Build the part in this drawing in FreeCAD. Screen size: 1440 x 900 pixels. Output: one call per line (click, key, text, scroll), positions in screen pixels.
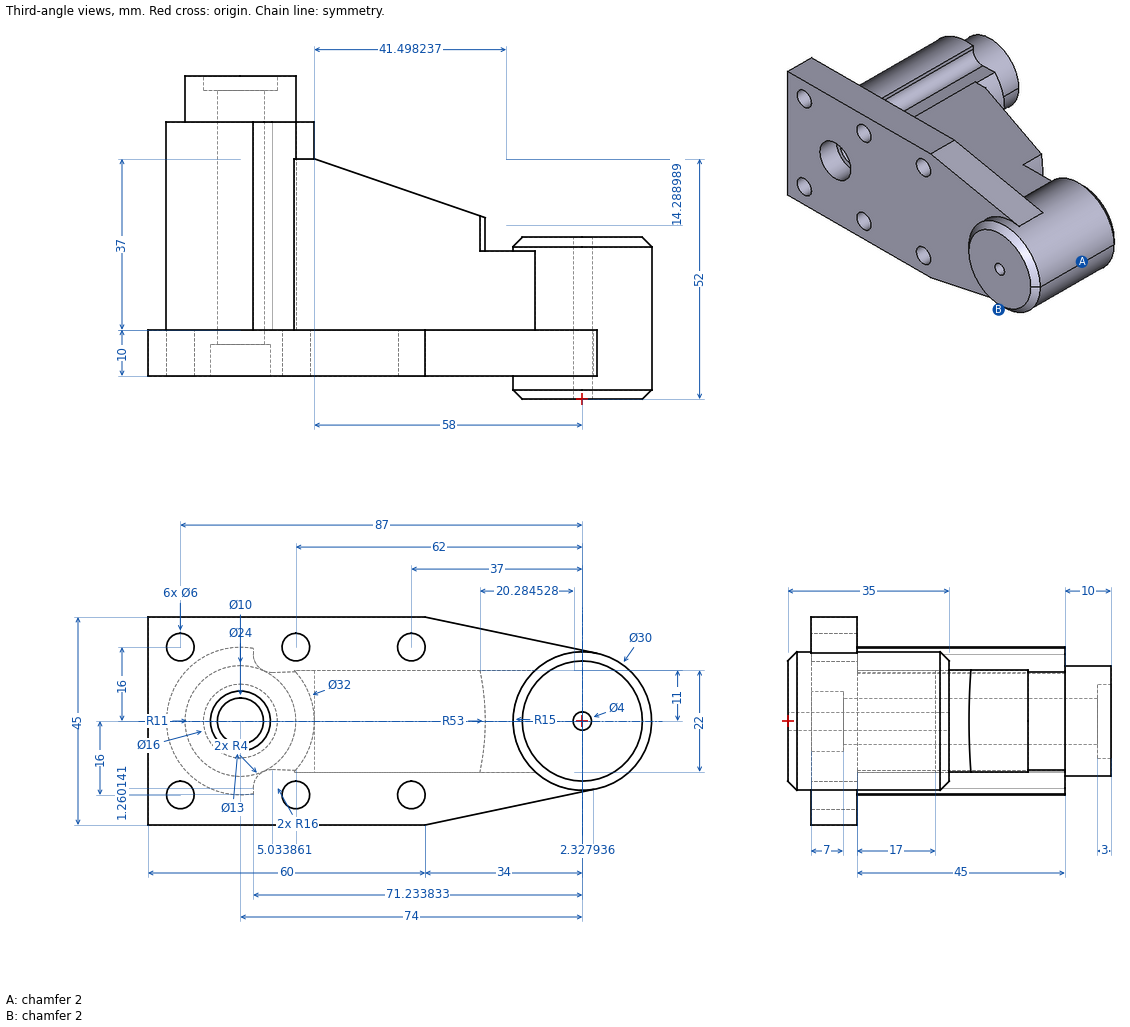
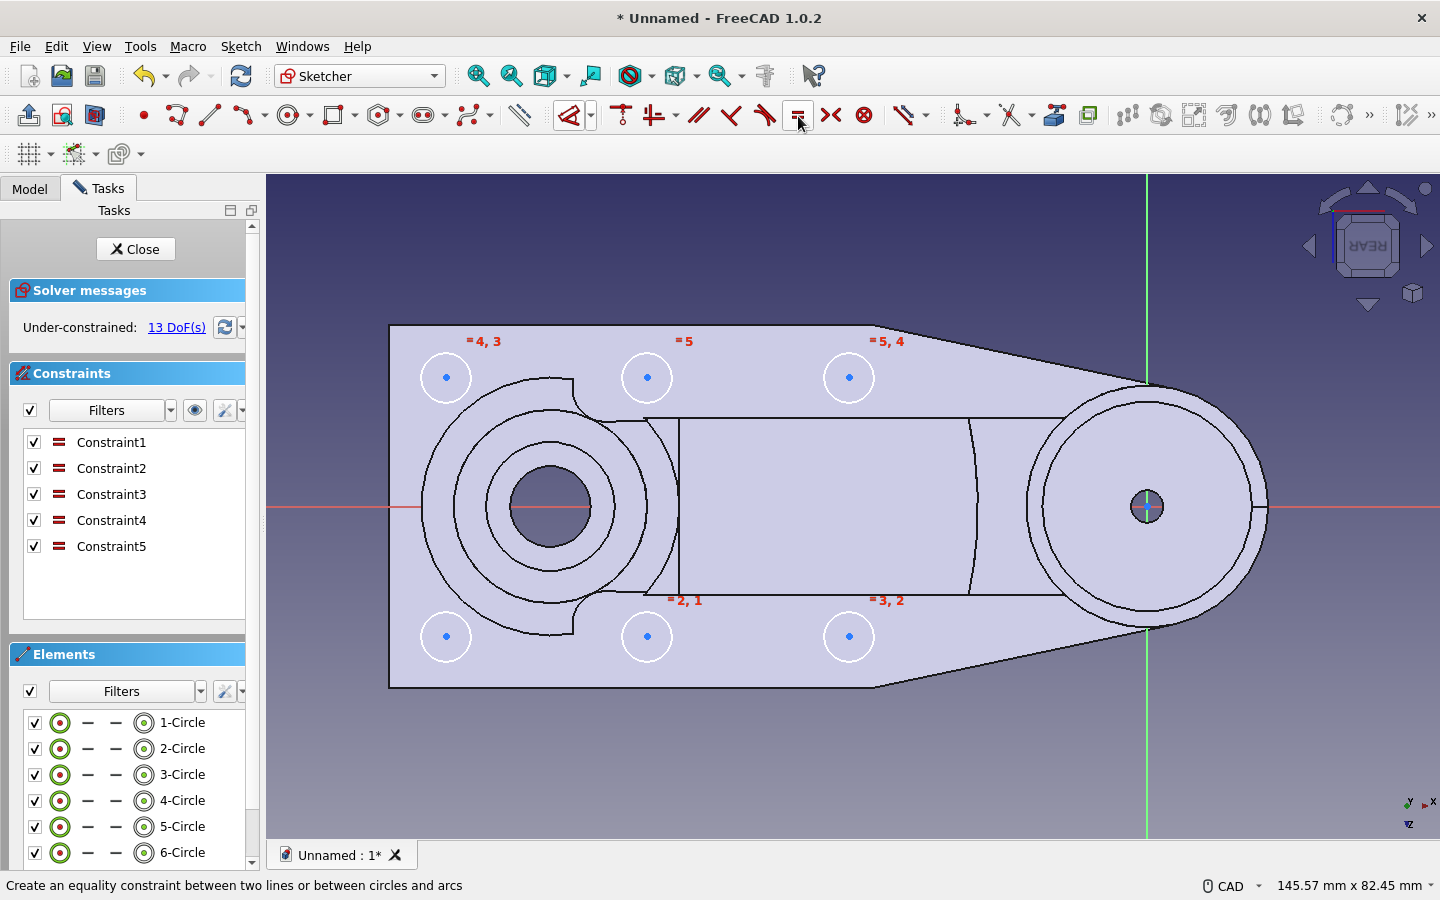
click(446, 637)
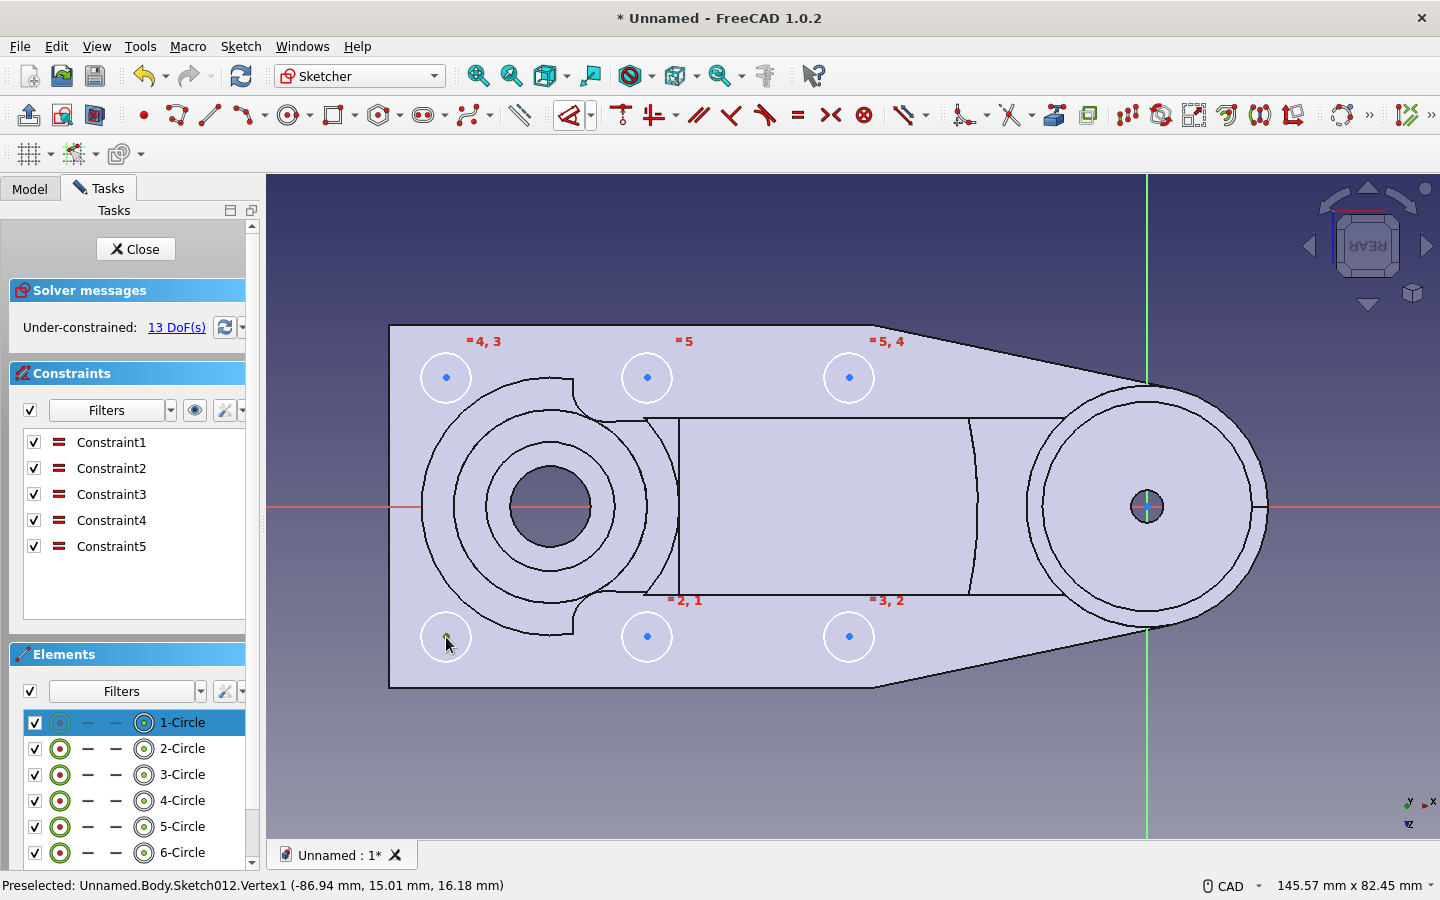
click(647, 637)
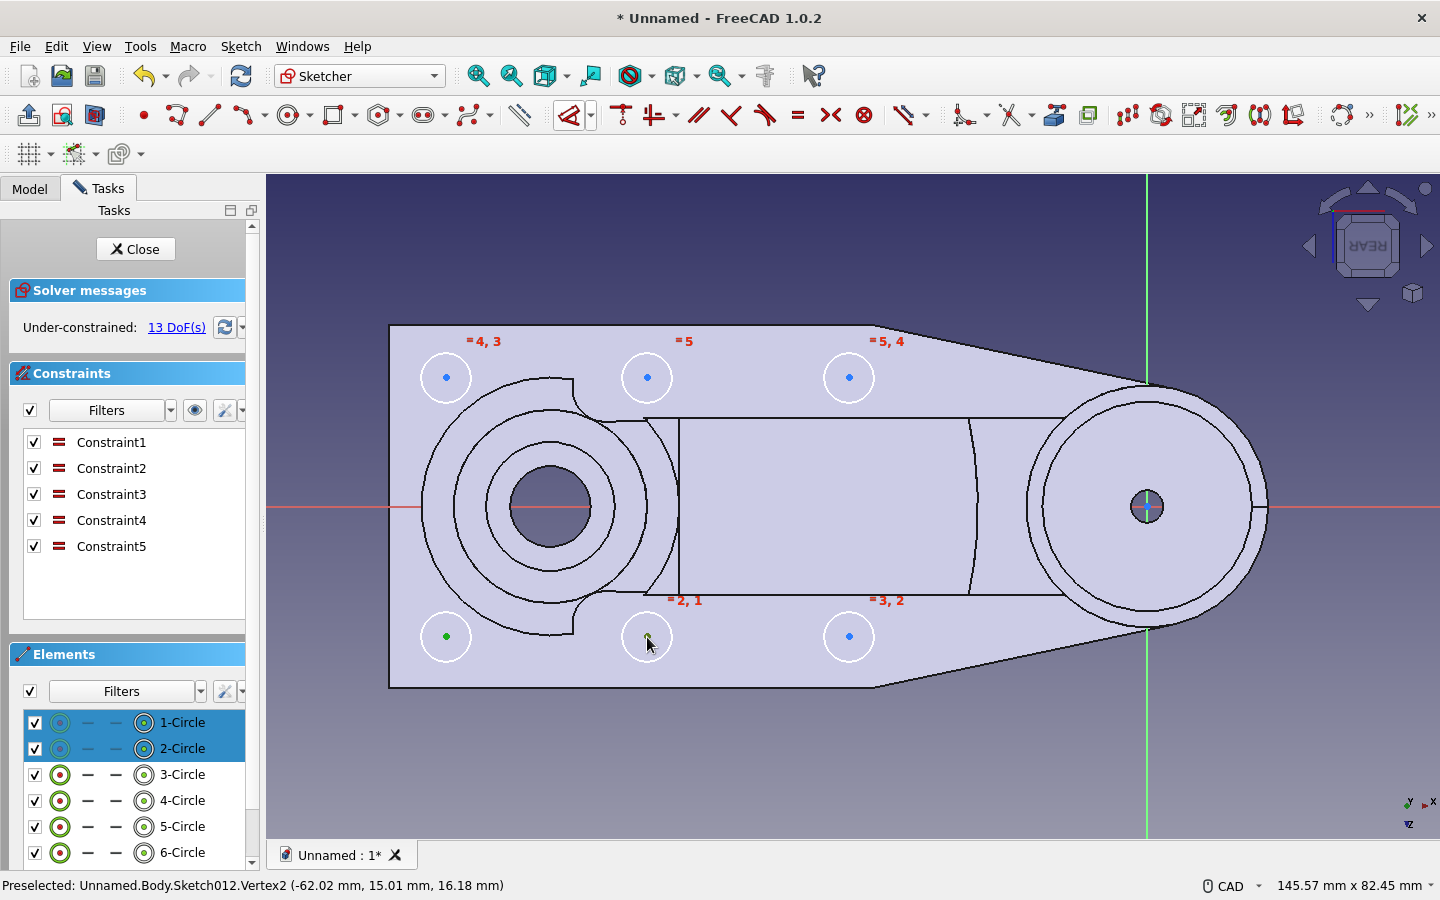
click(676, 116)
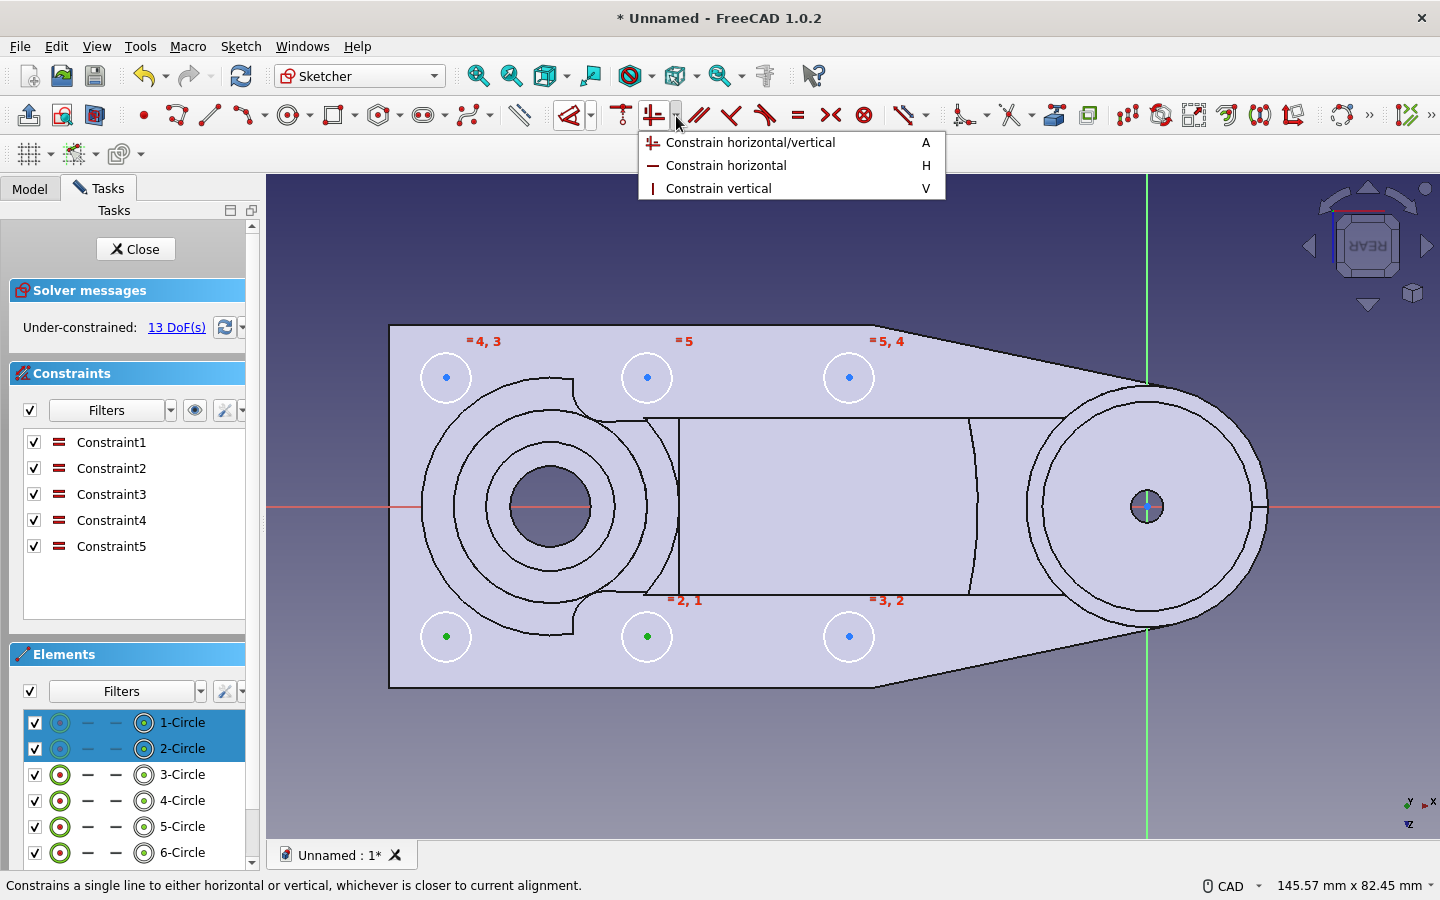
click(792, 166)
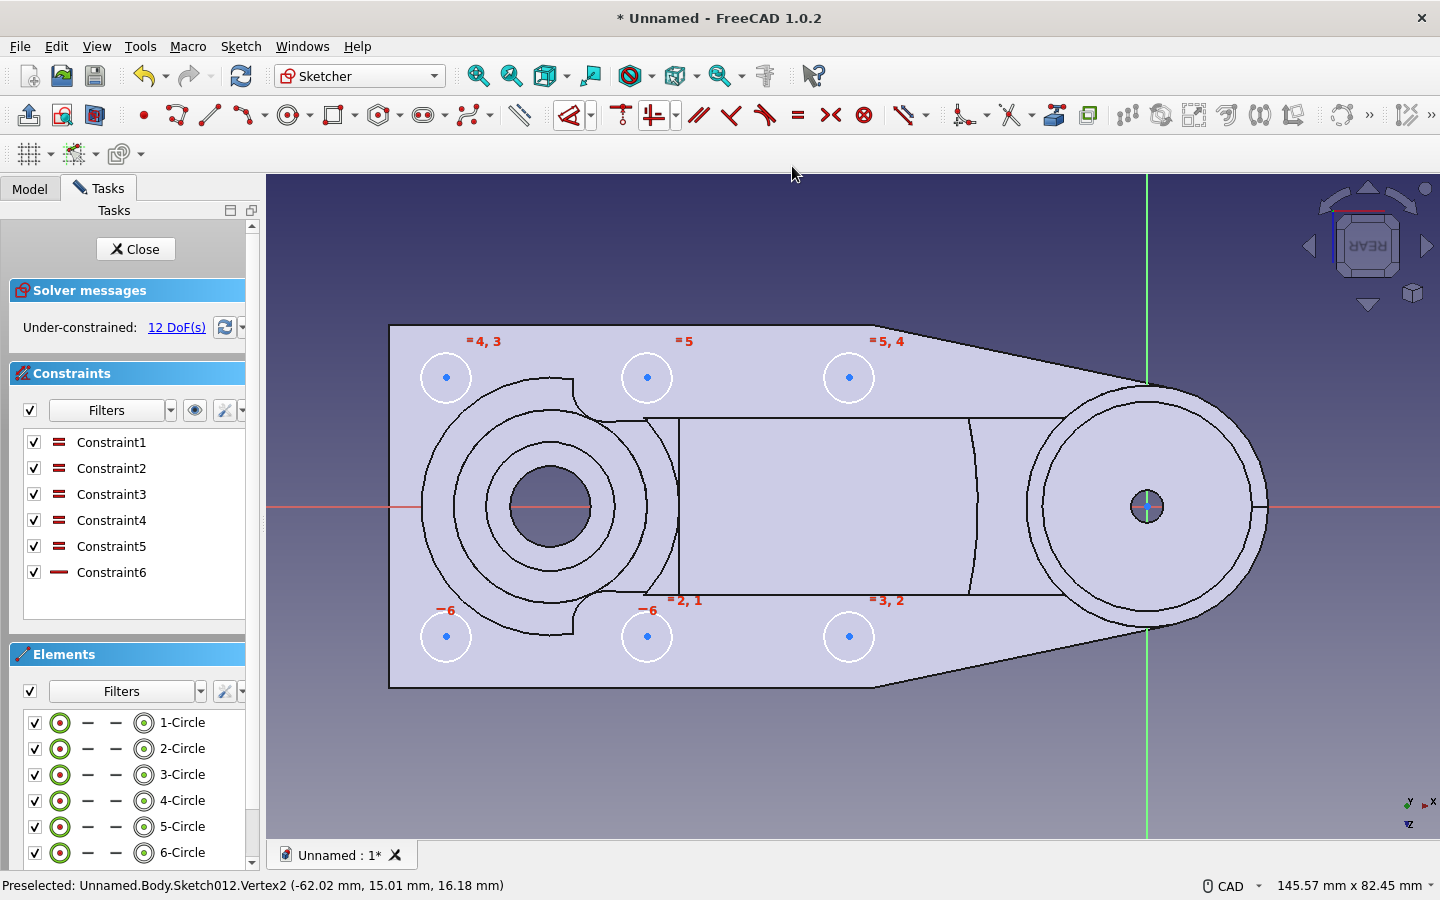
click(647, 637)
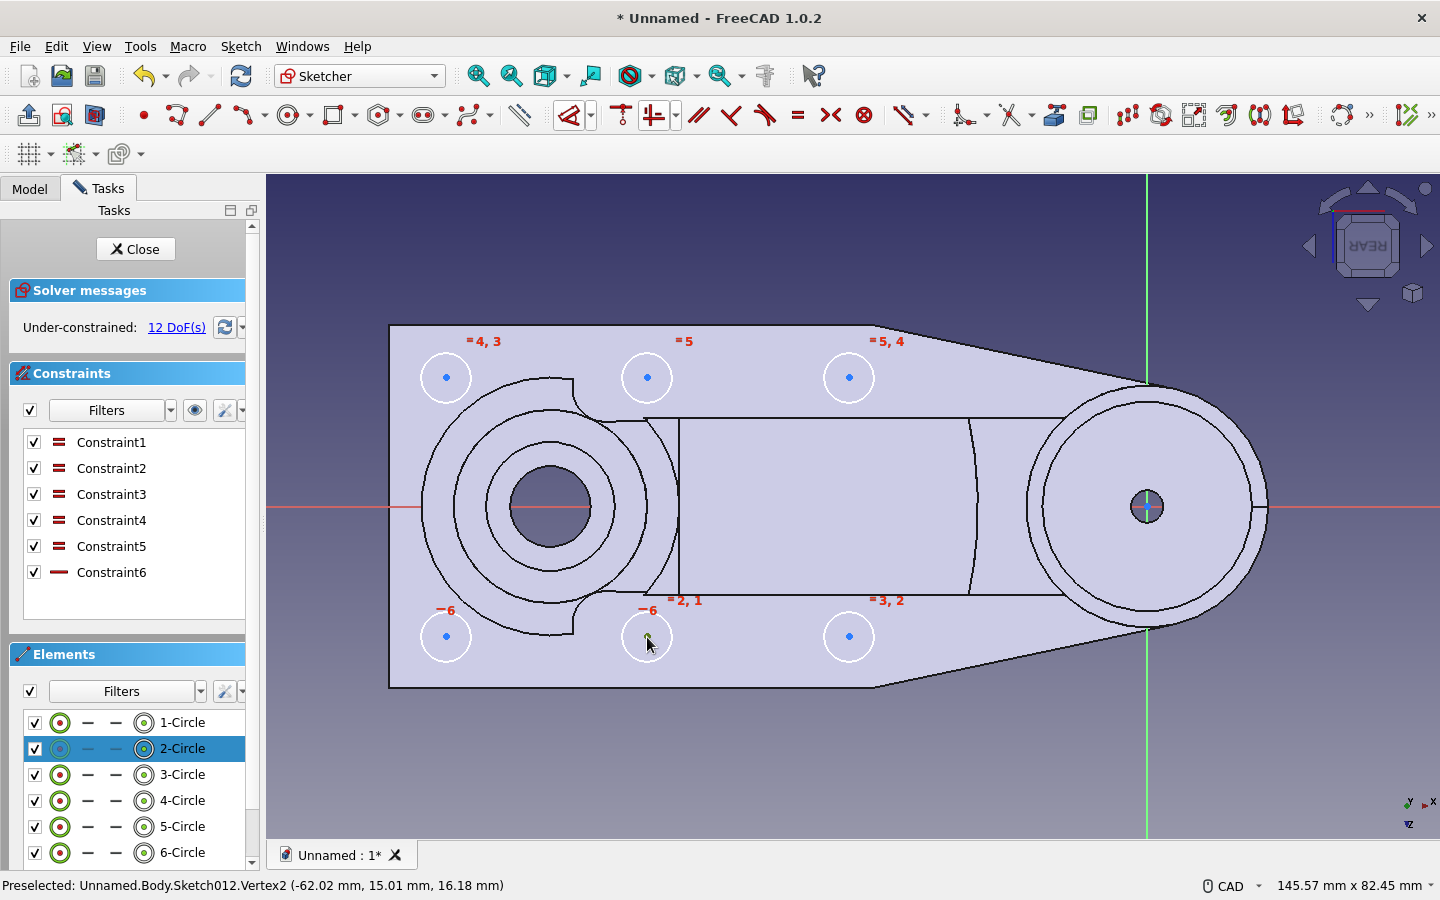
click(849, 637)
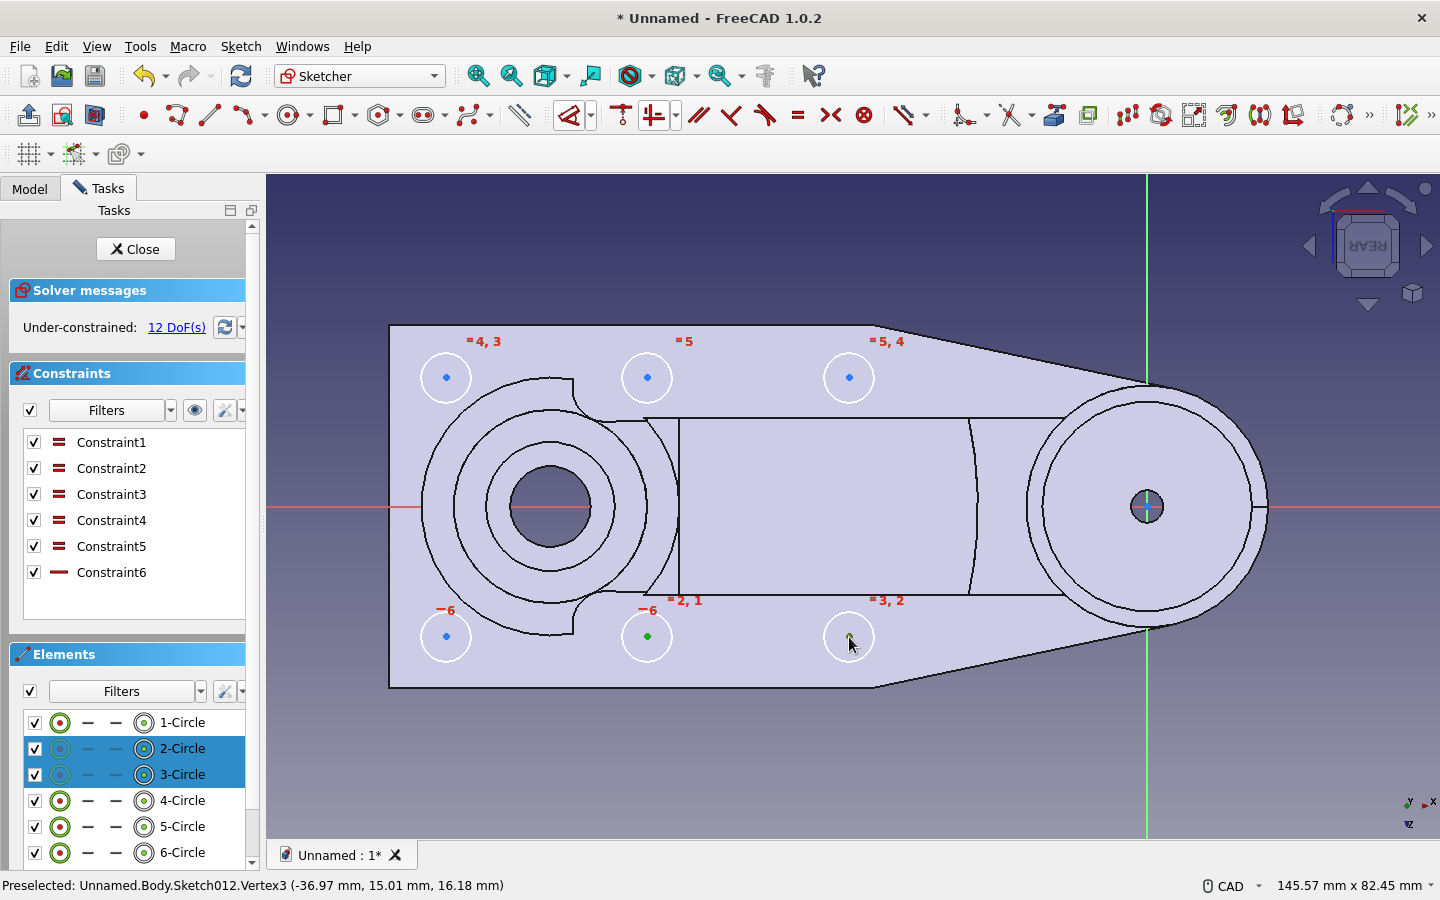
key(h)